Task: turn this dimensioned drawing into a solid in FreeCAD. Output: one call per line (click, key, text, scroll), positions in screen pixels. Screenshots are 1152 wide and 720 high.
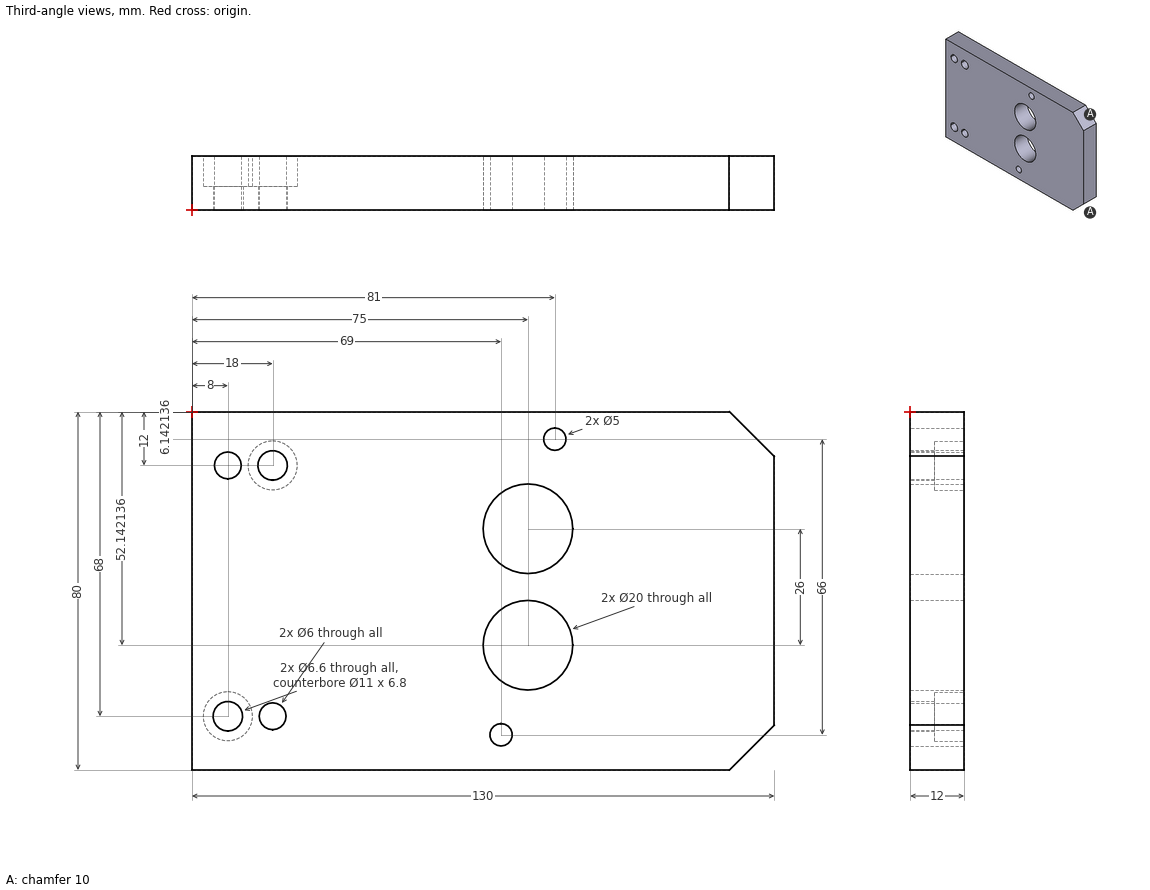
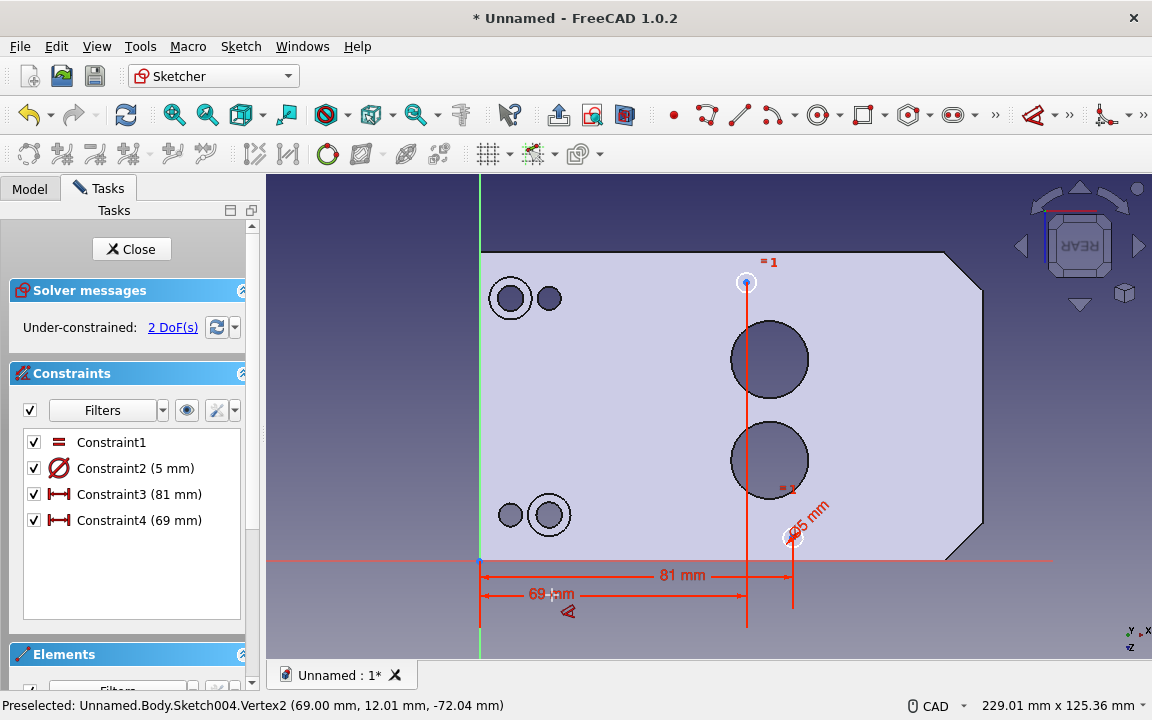
click(793, 538)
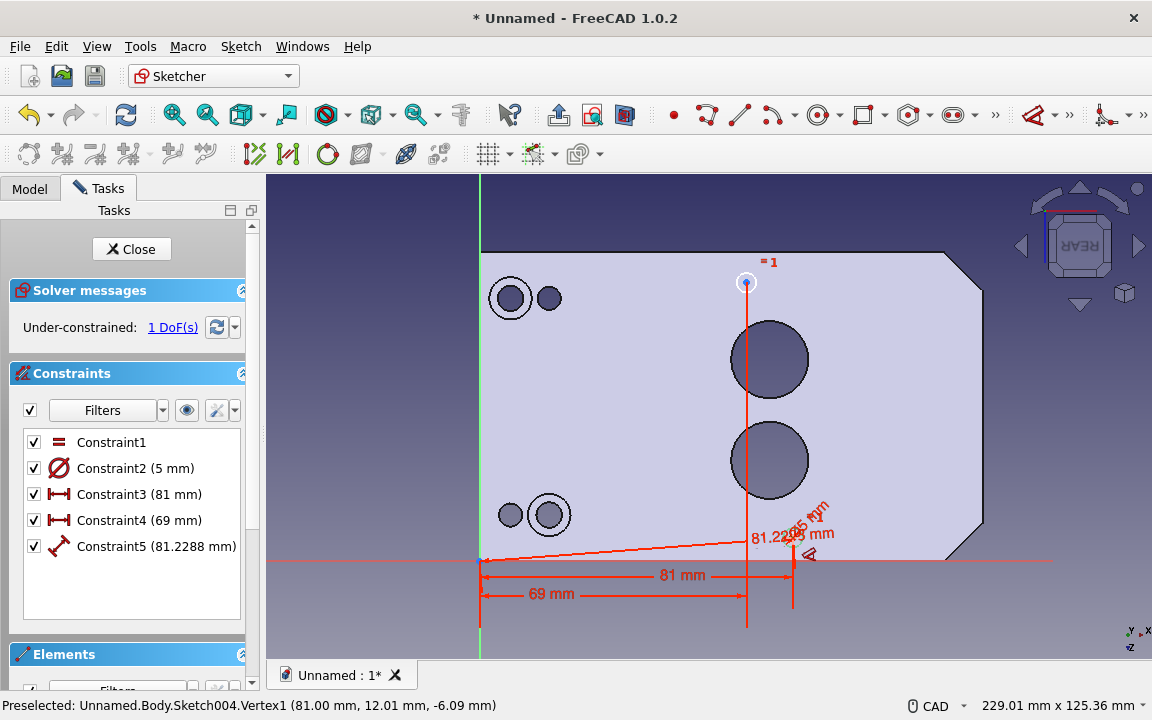
click(747, 283)
click(827, 410)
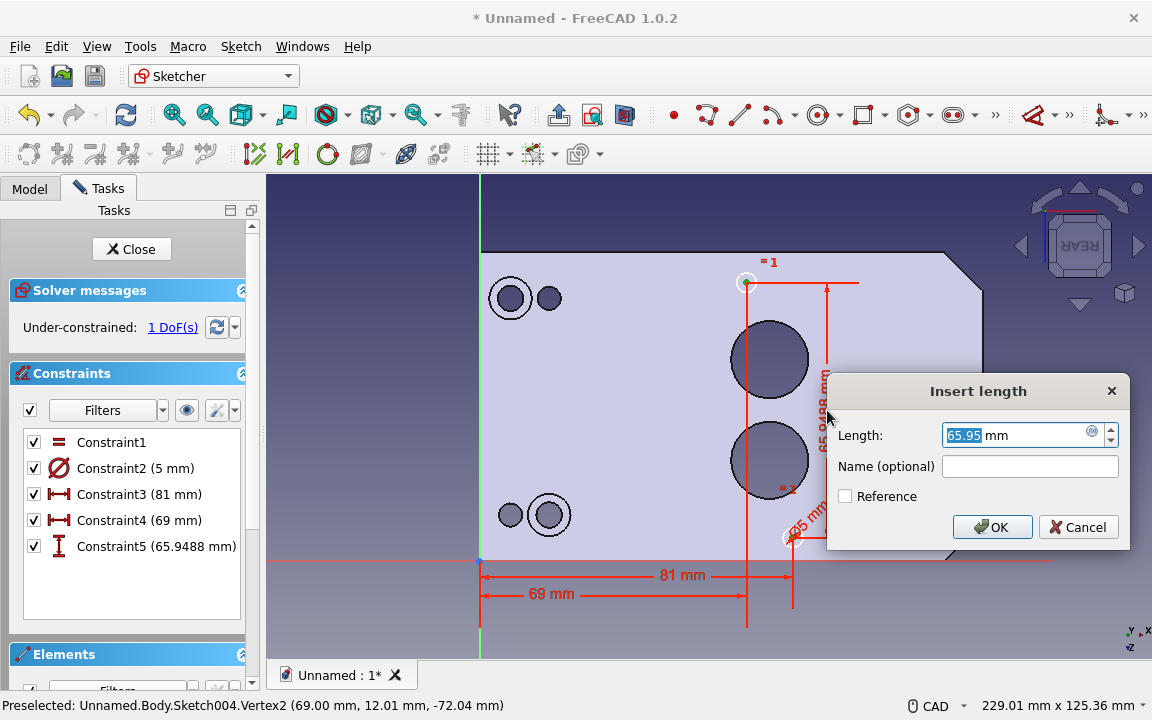
text(66)
key(Return)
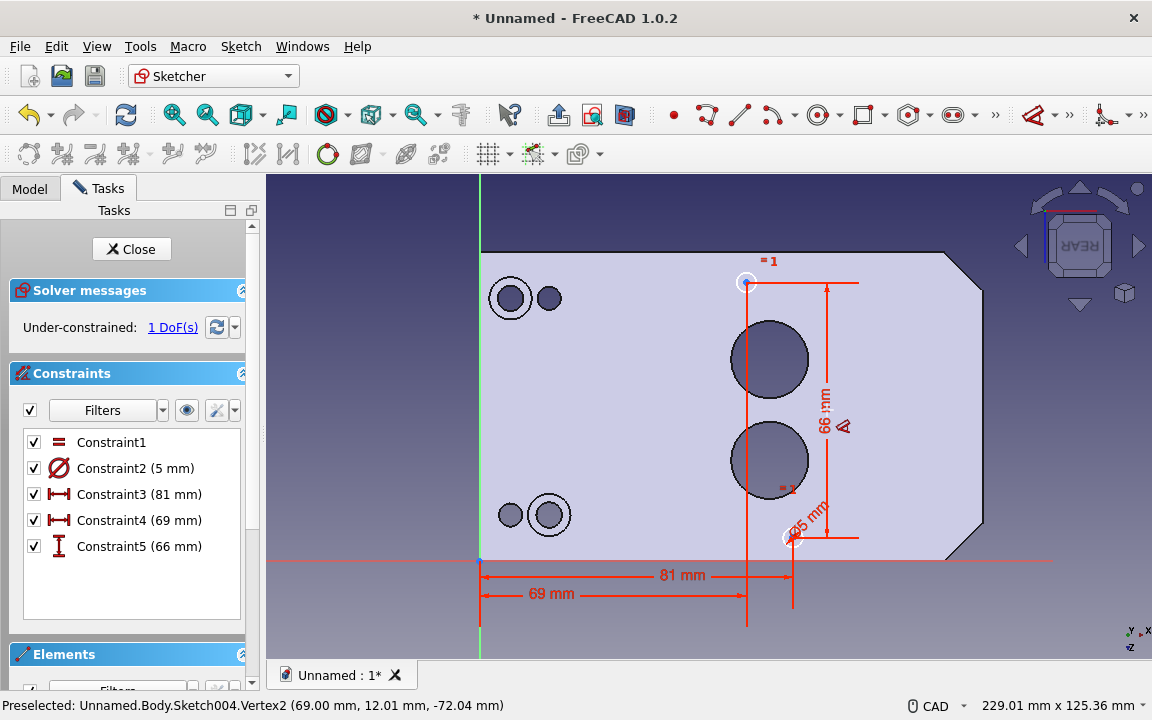
scroll(793, 538, up, 3)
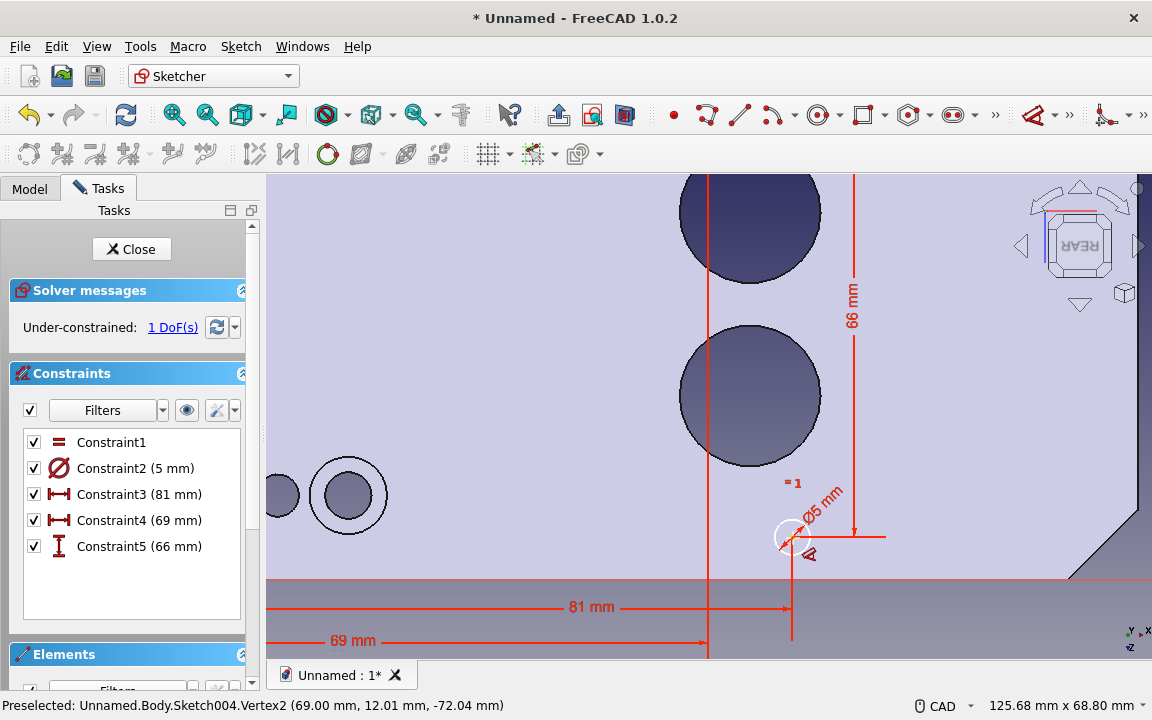
click(792, 537)
click(826, 559)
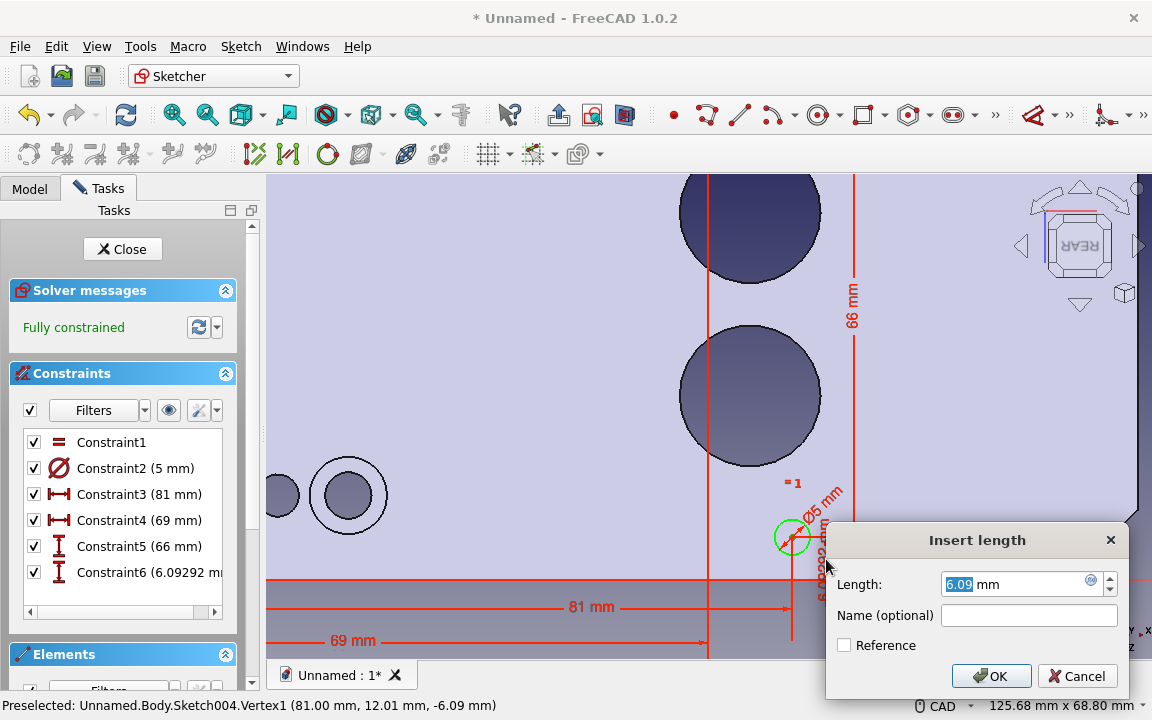
text(6.142136)
key(Return)
key(Escape)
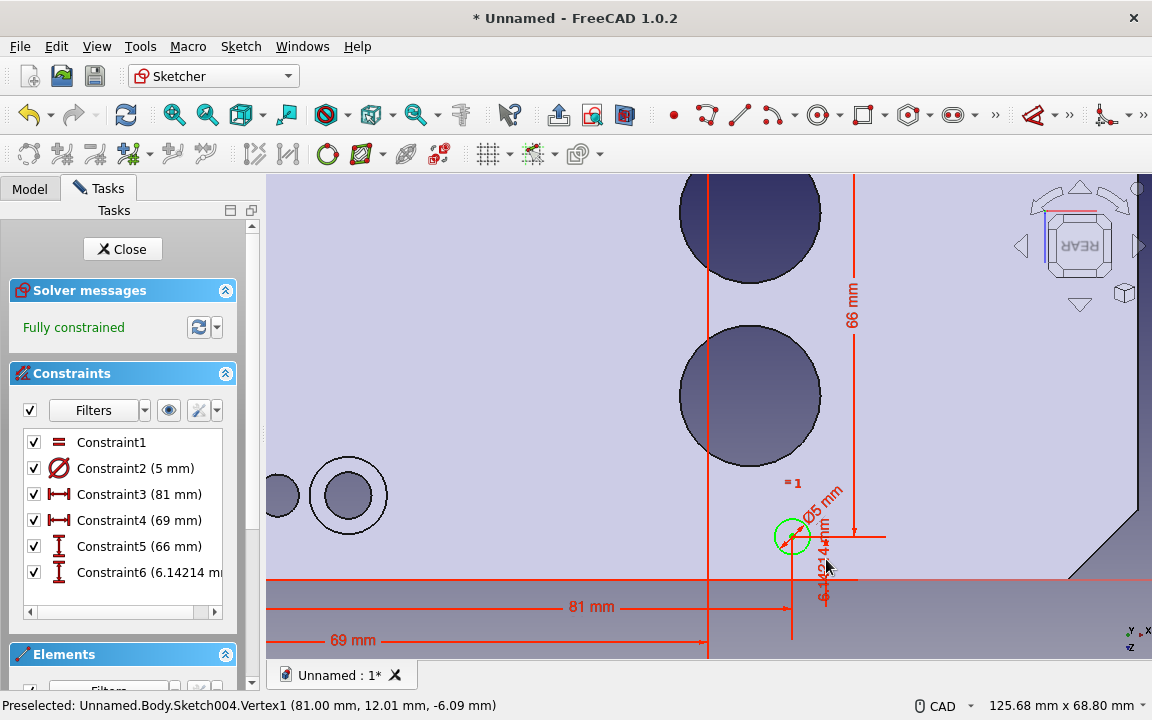
click(123, 249)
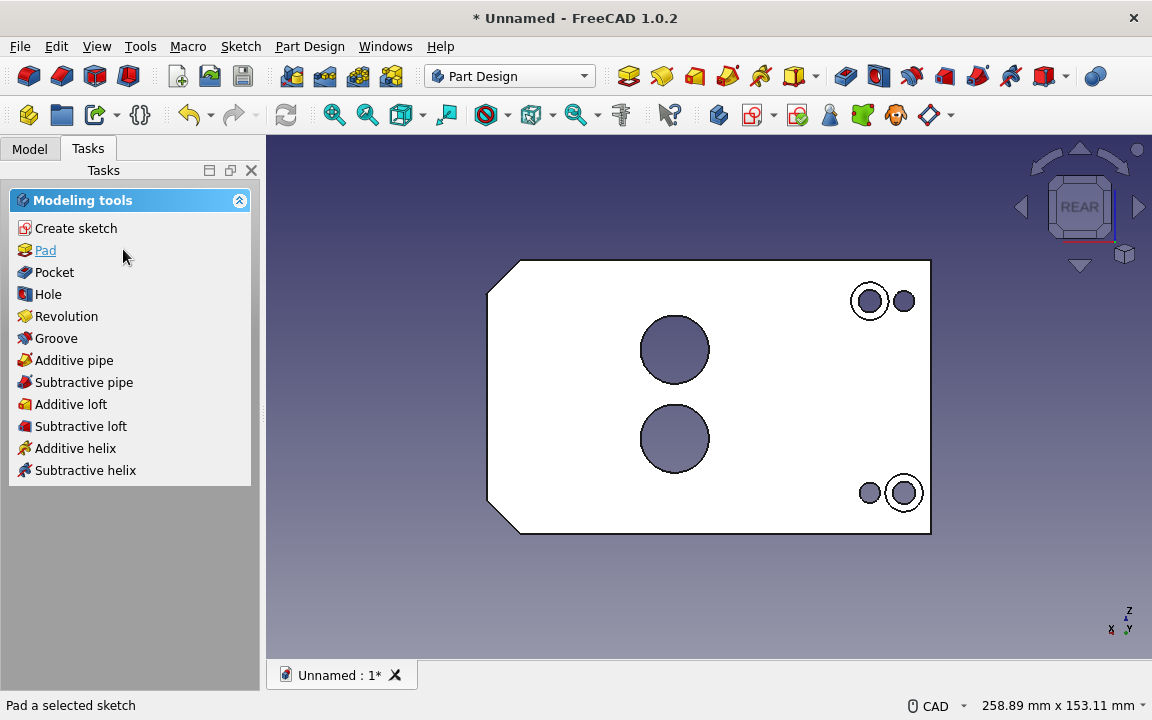
click(846, 76)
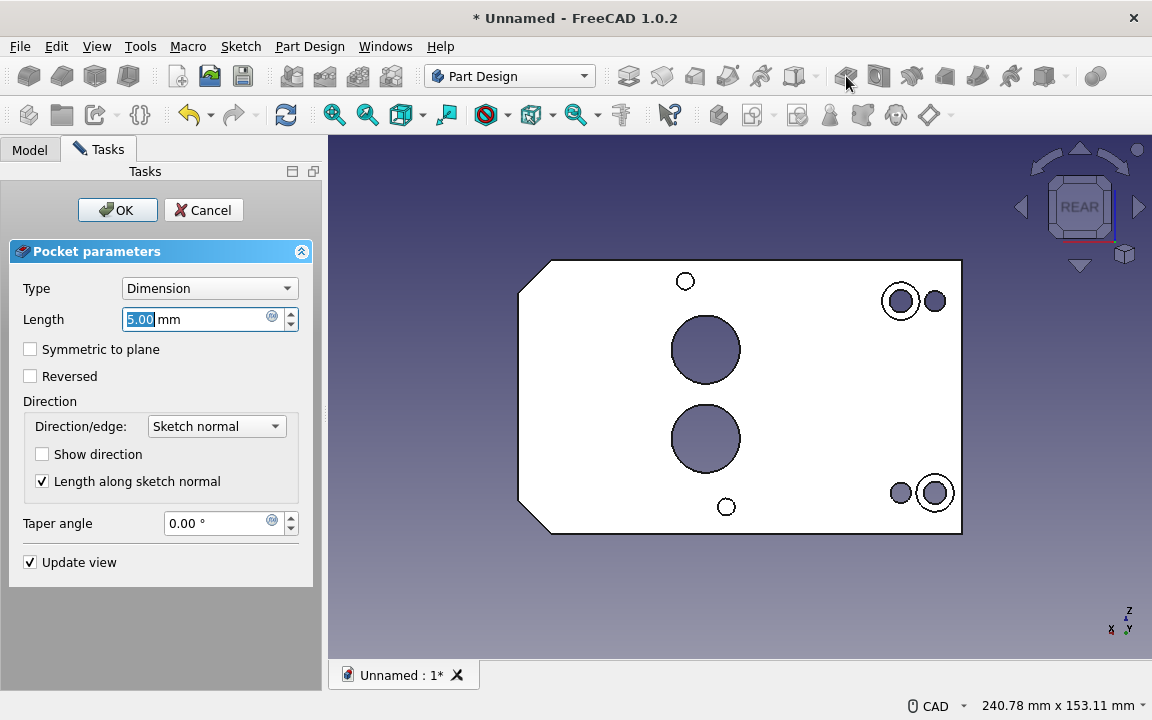
click(210, 288)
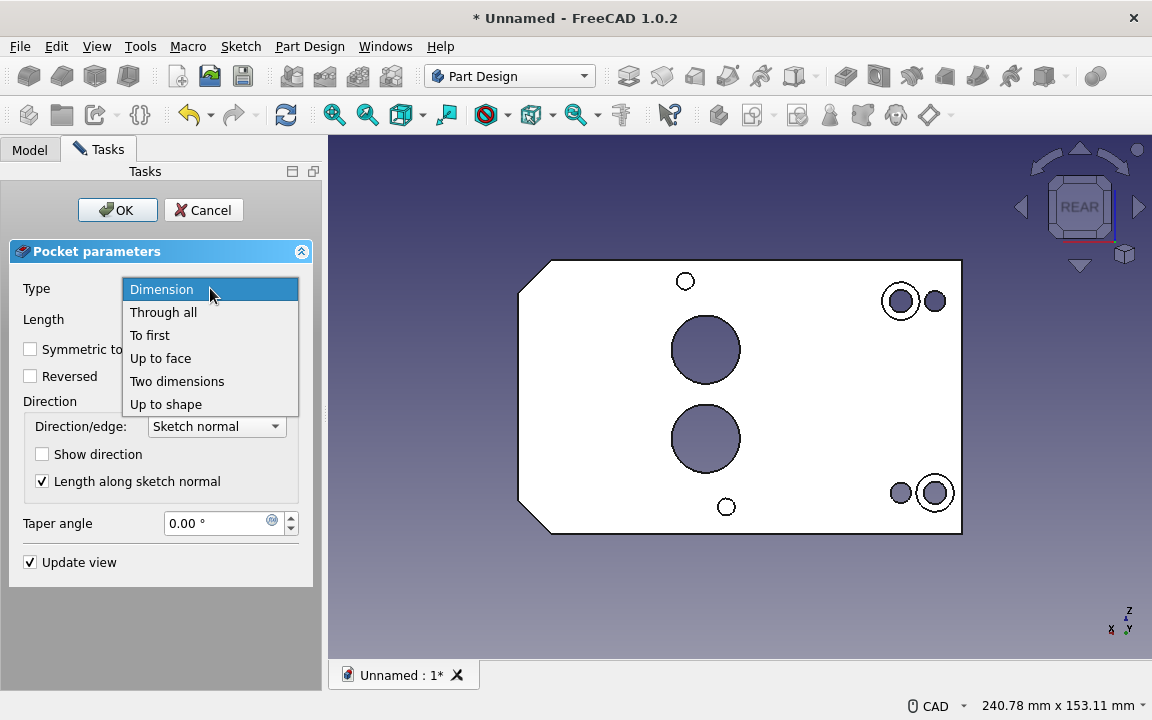
click(208, 312)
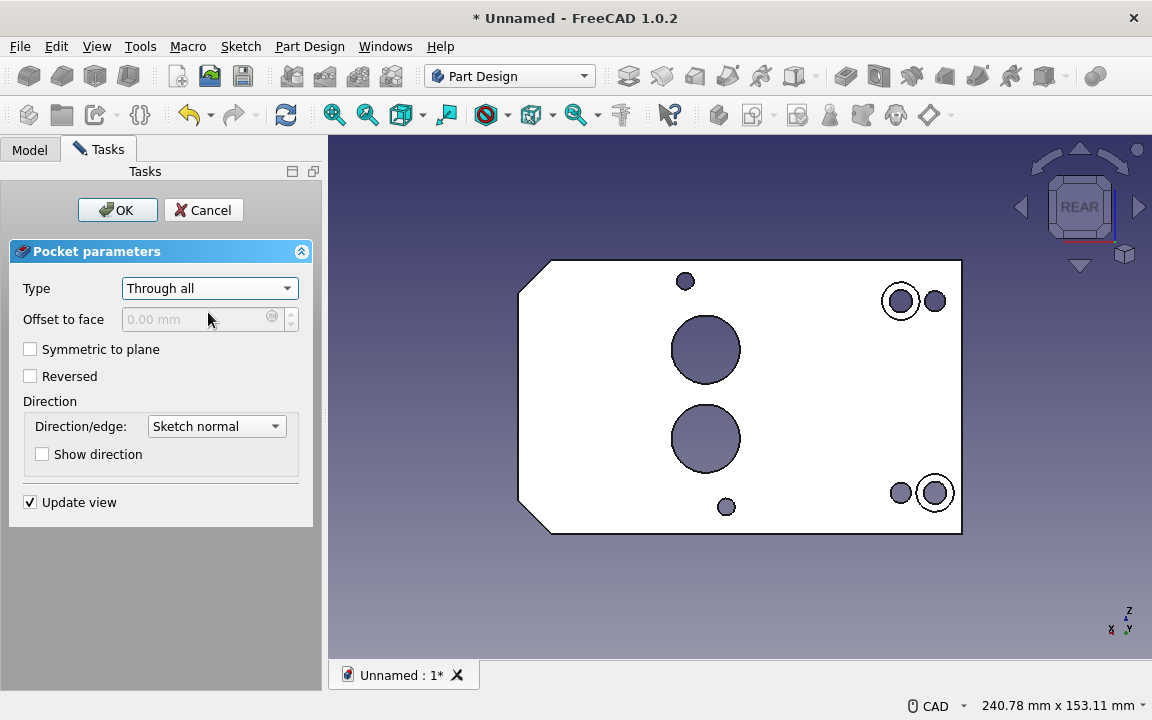
click(118, 210)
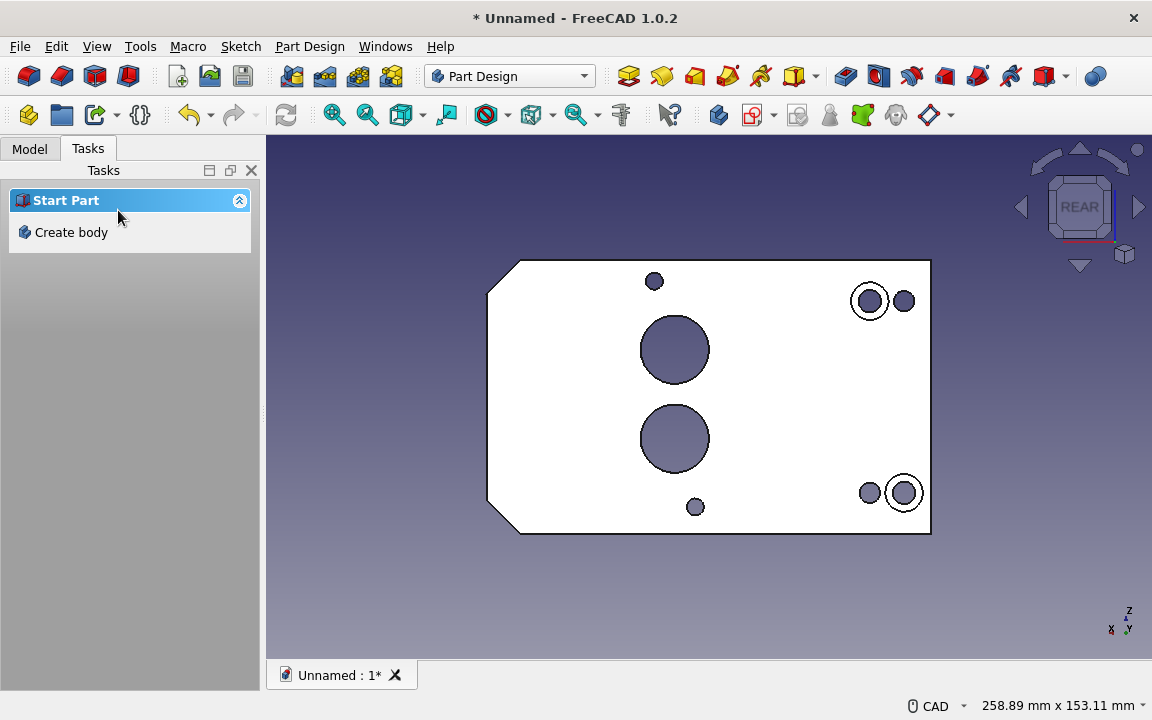
key(0)